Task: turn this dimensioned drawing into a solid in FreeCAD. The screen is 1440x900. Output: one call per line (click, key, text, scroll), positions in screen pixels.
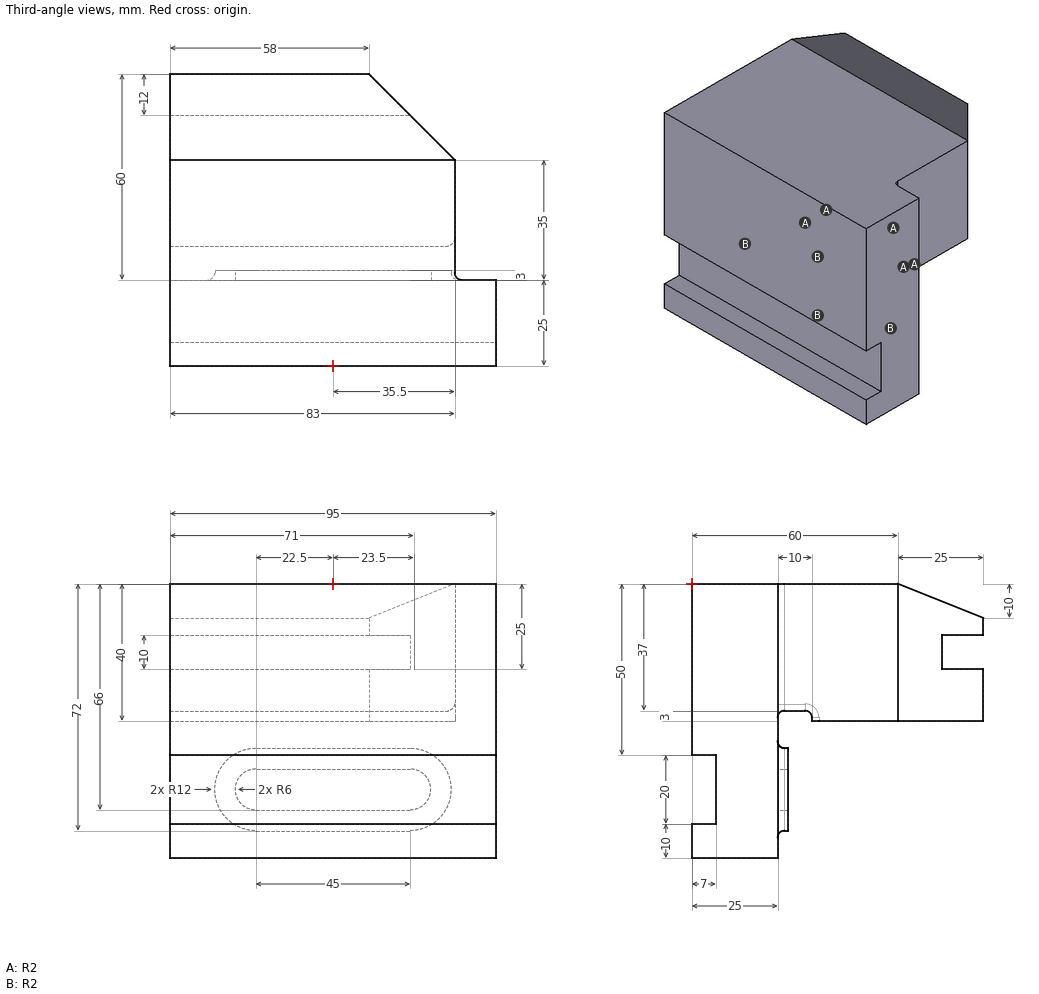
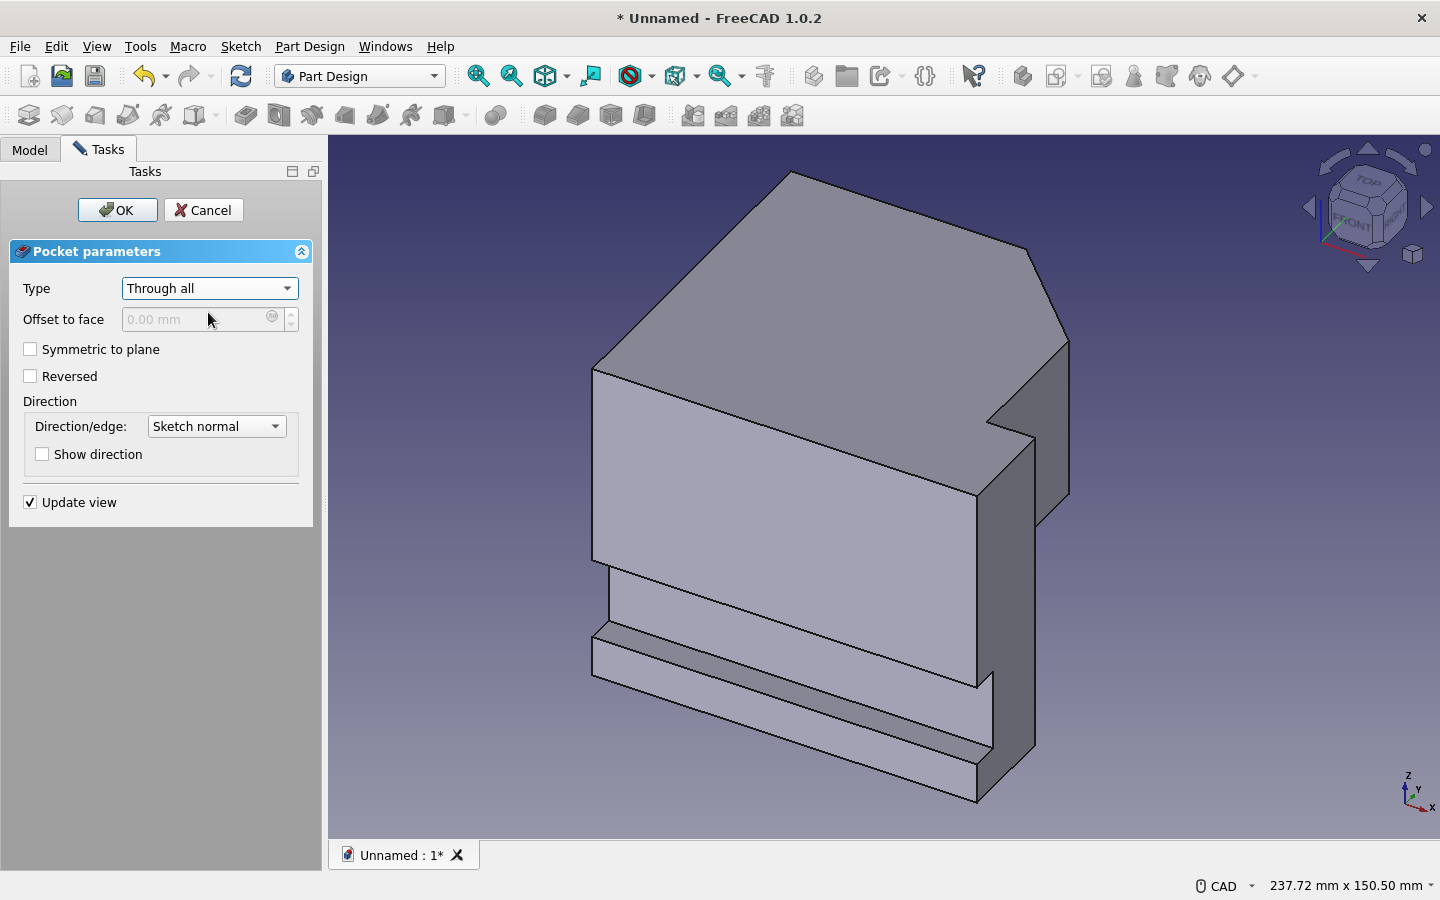
click(118, 210)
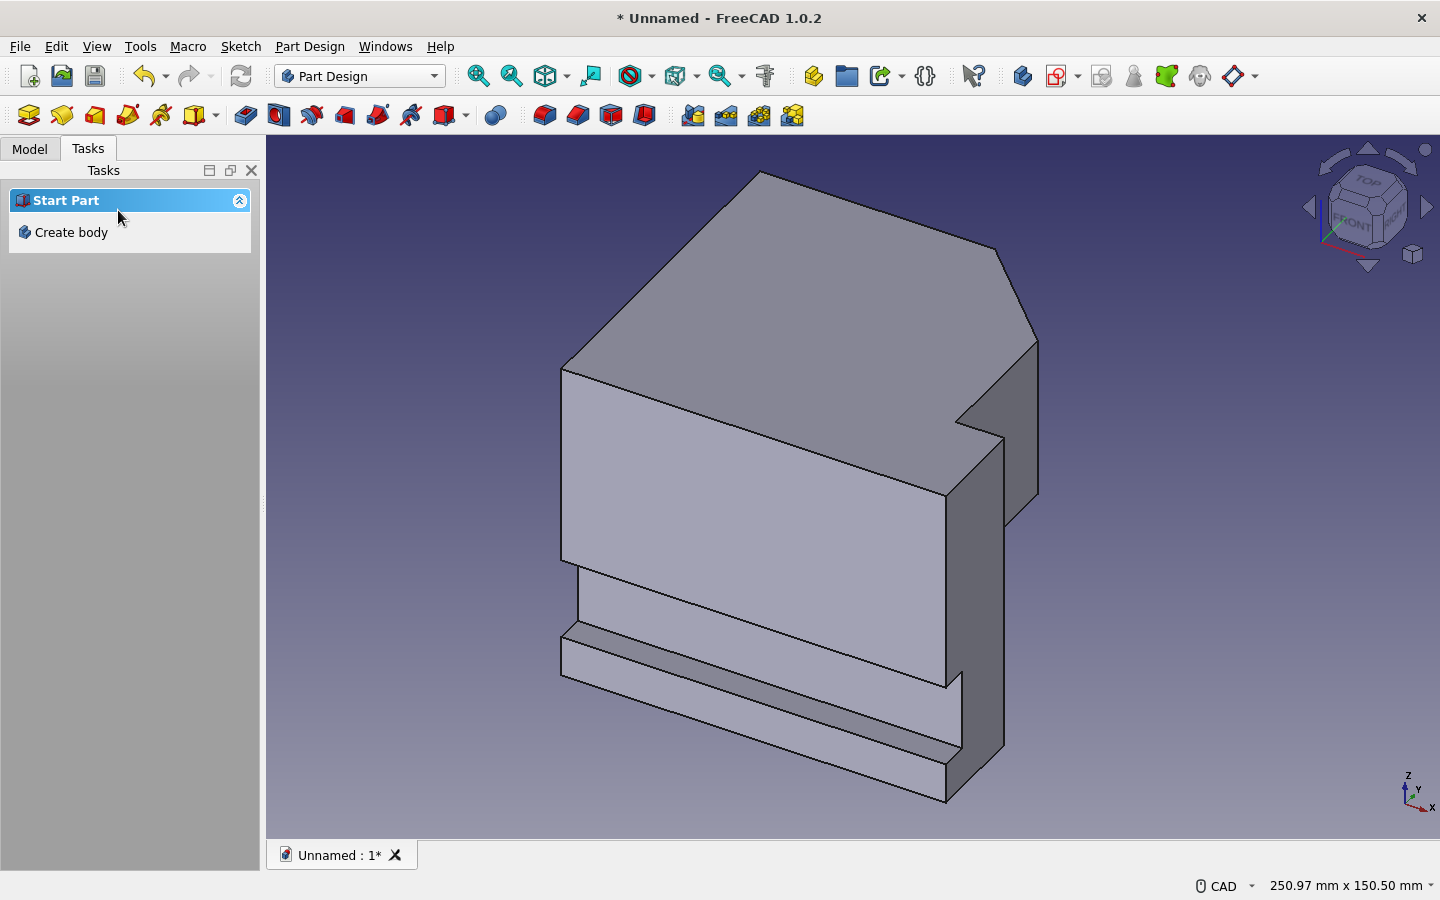
key(0)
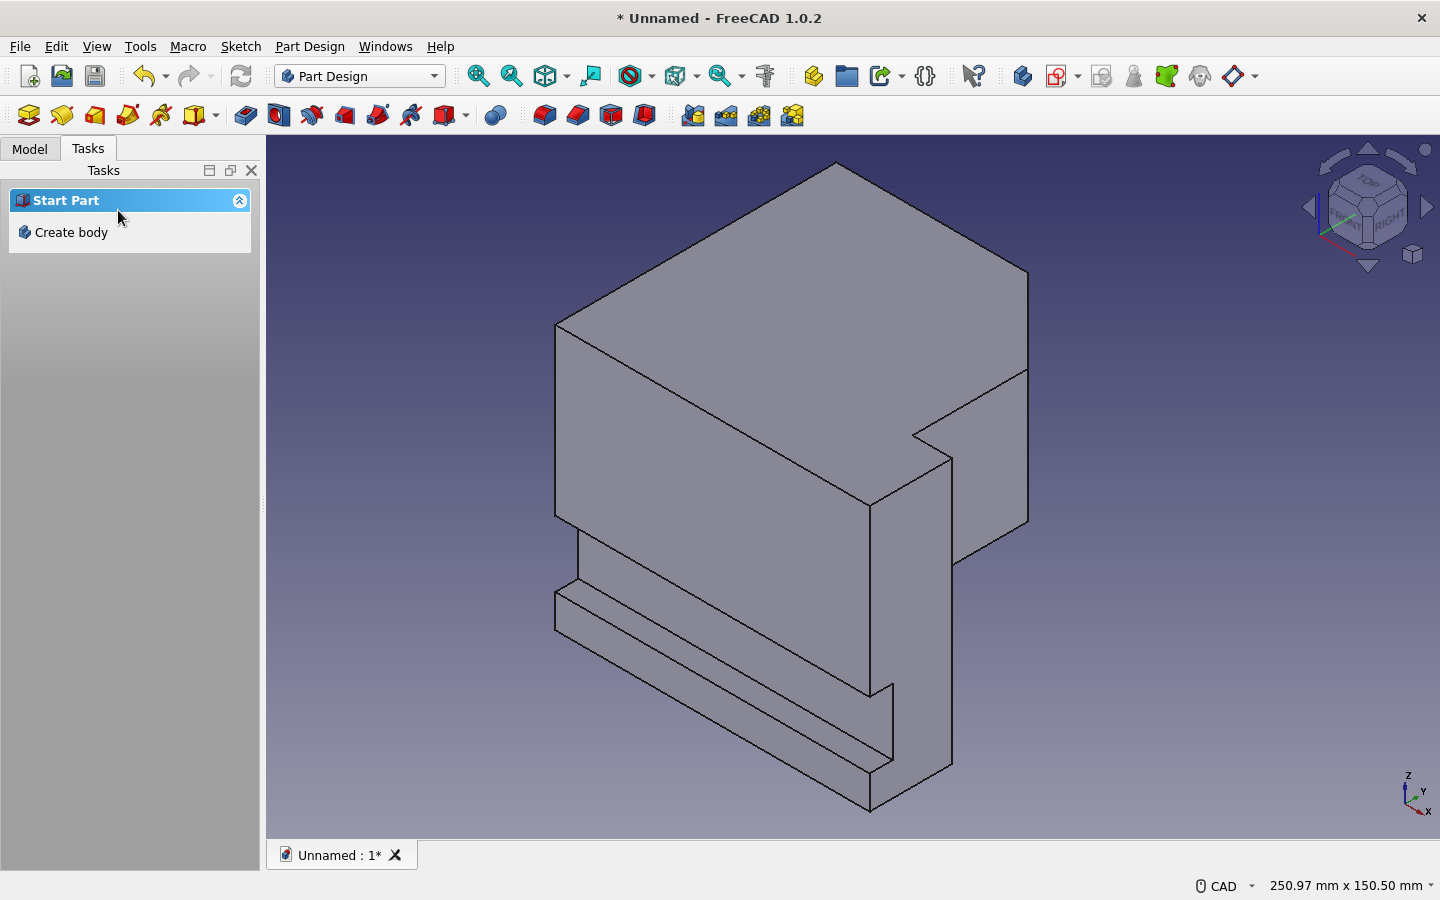
key(2)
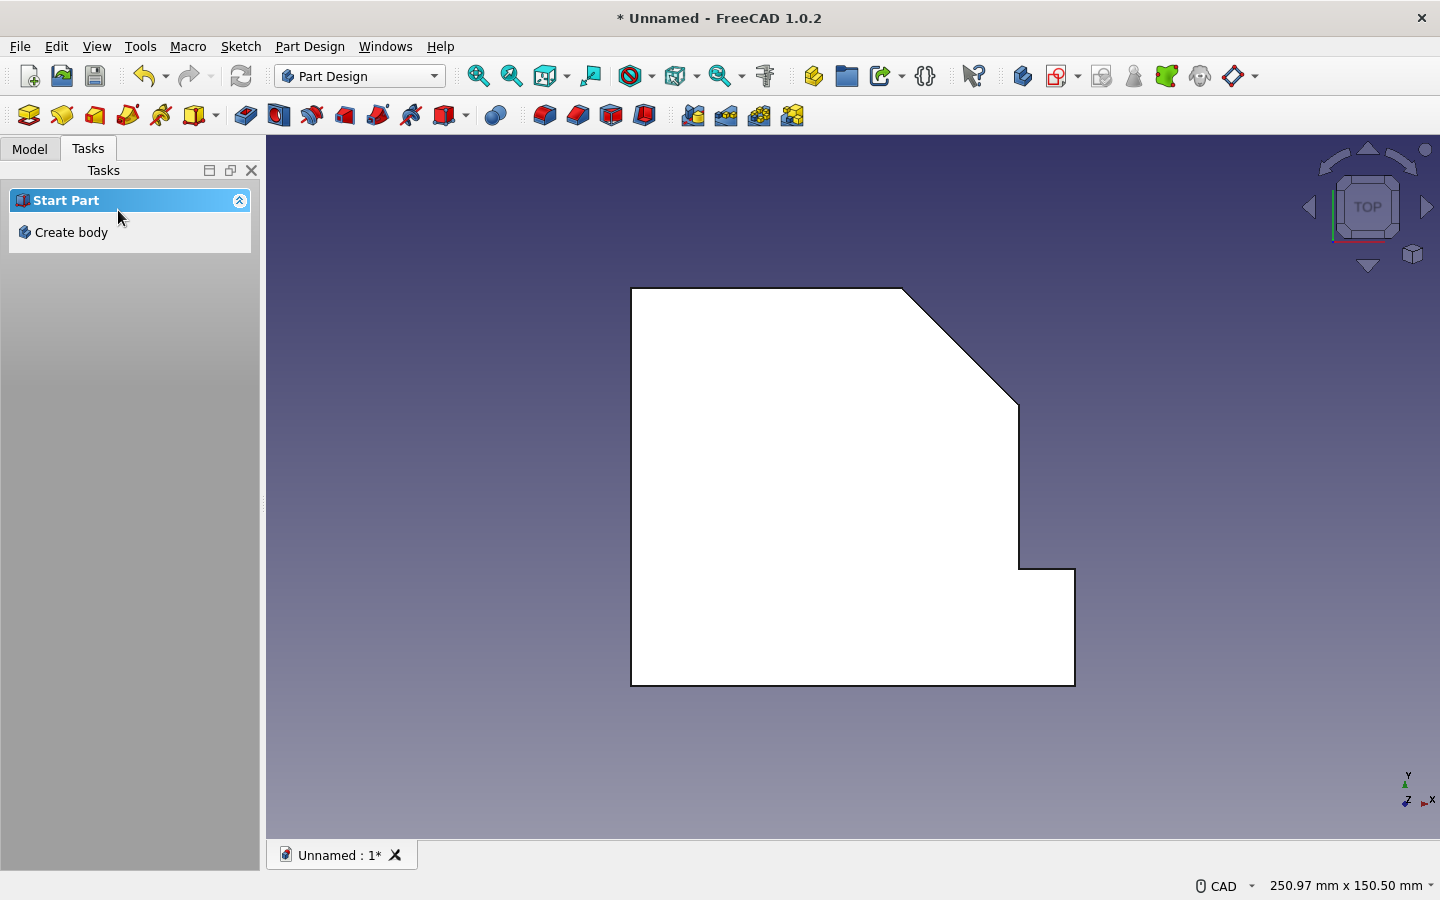
key(1)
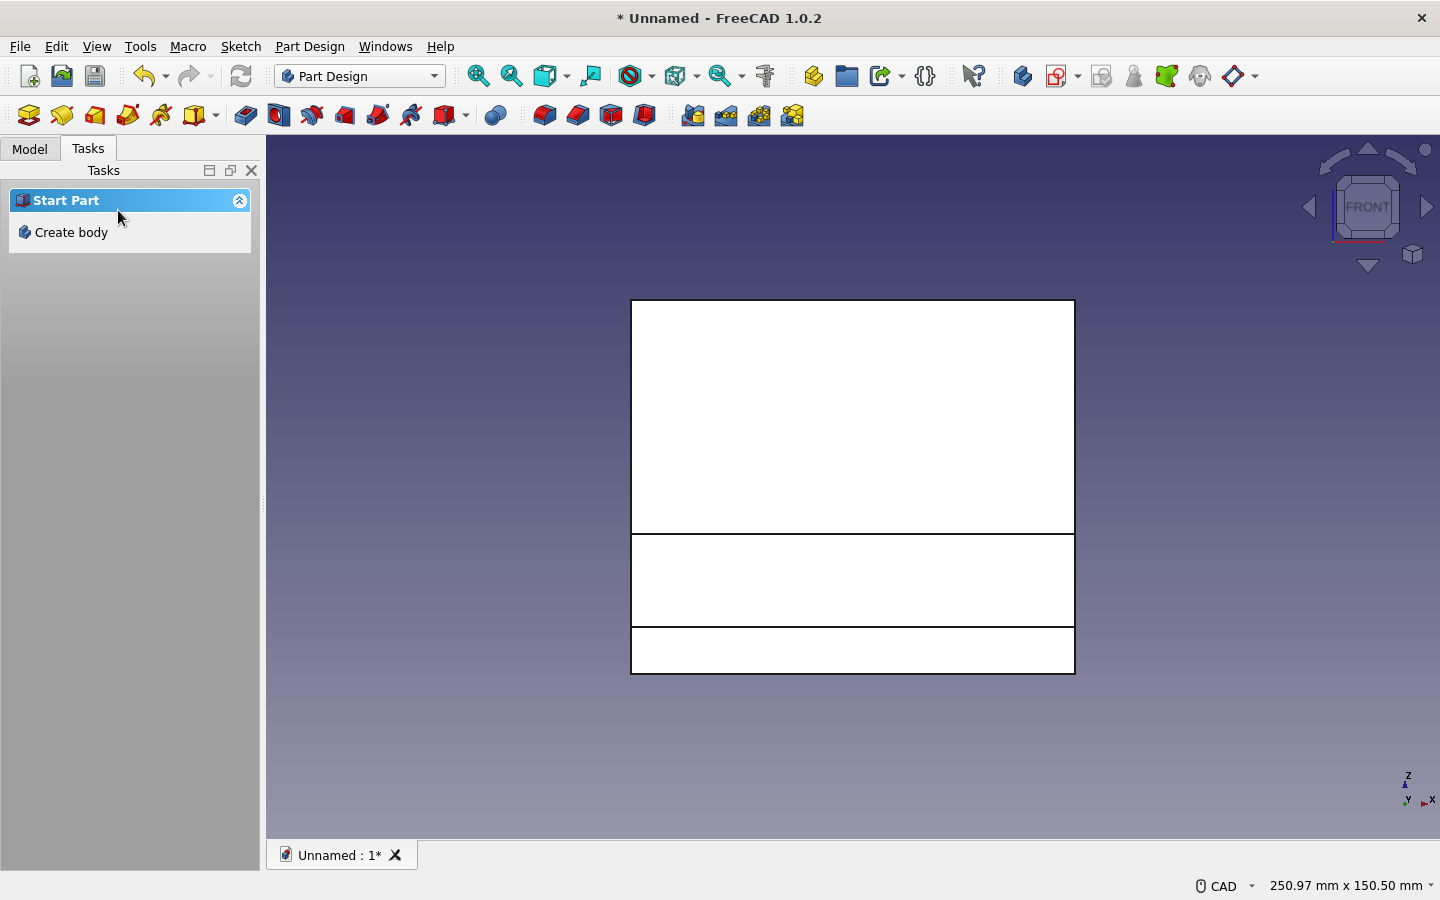
key(3)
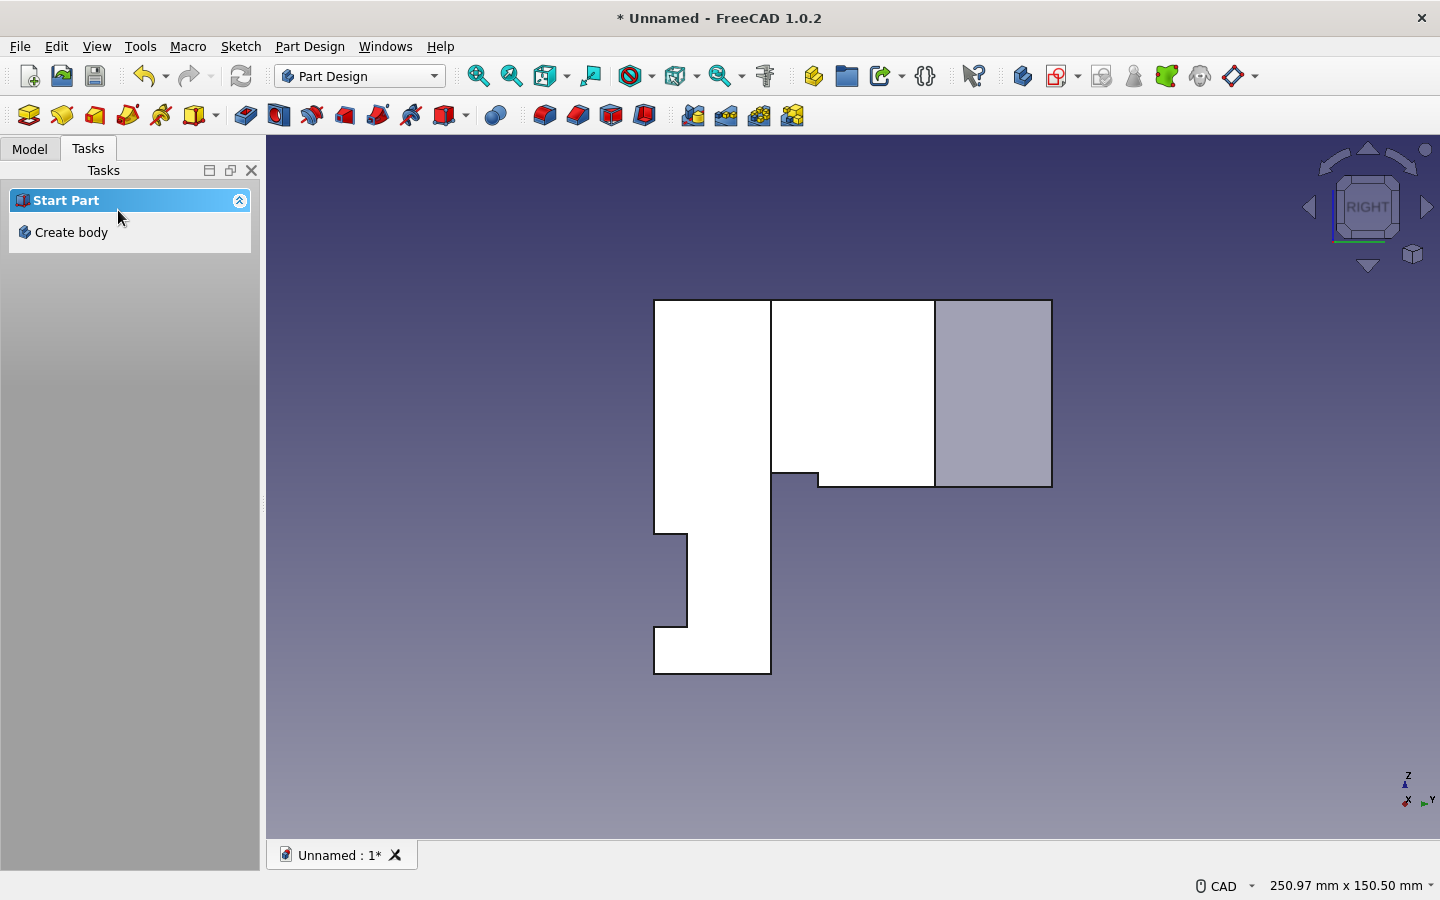
click(818, 479)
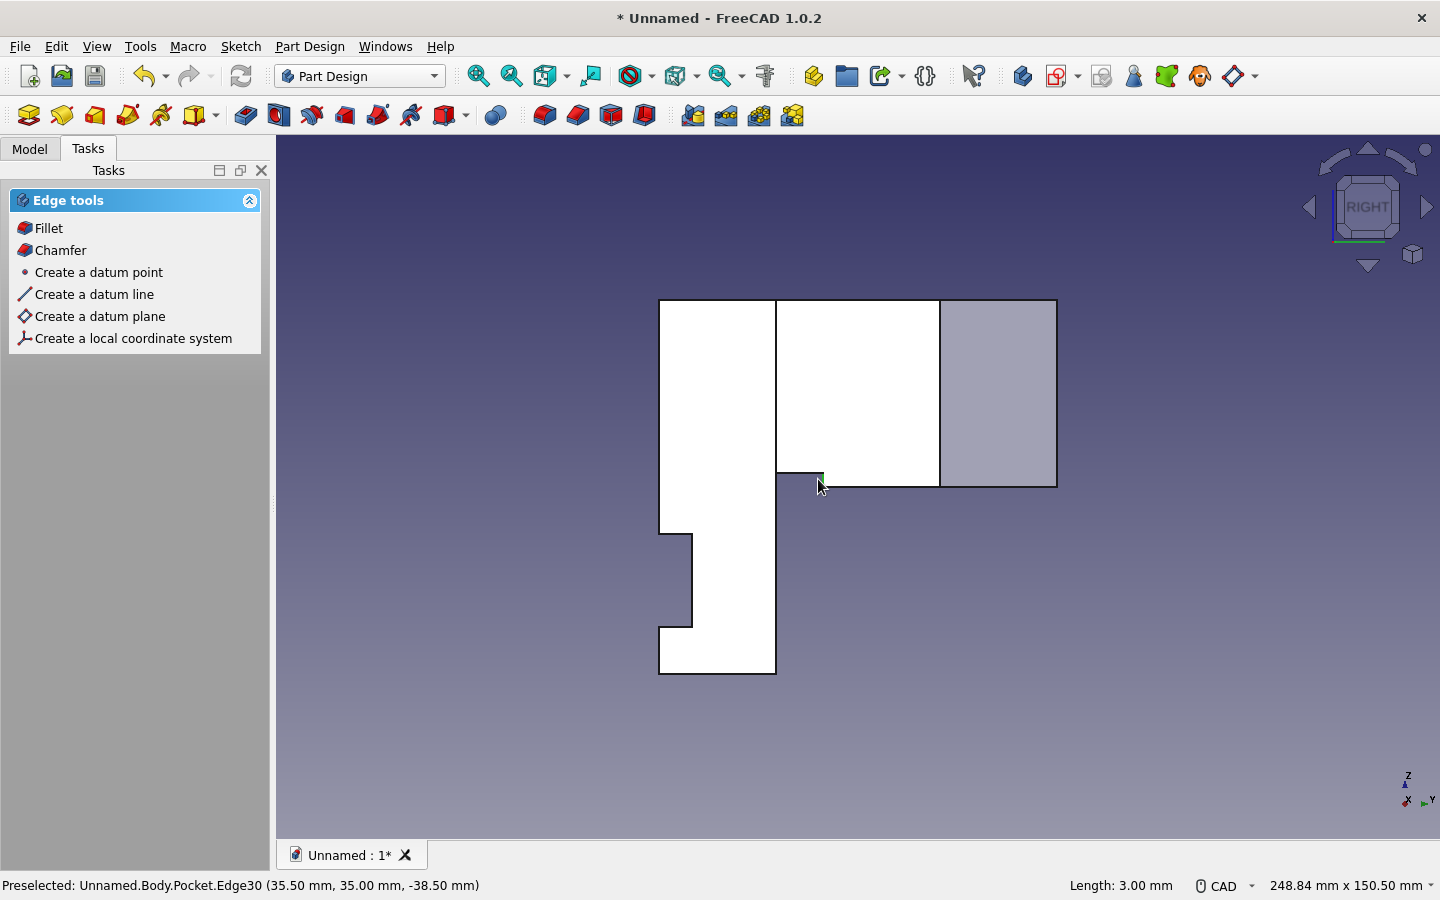
click(800, 472, ctrl)